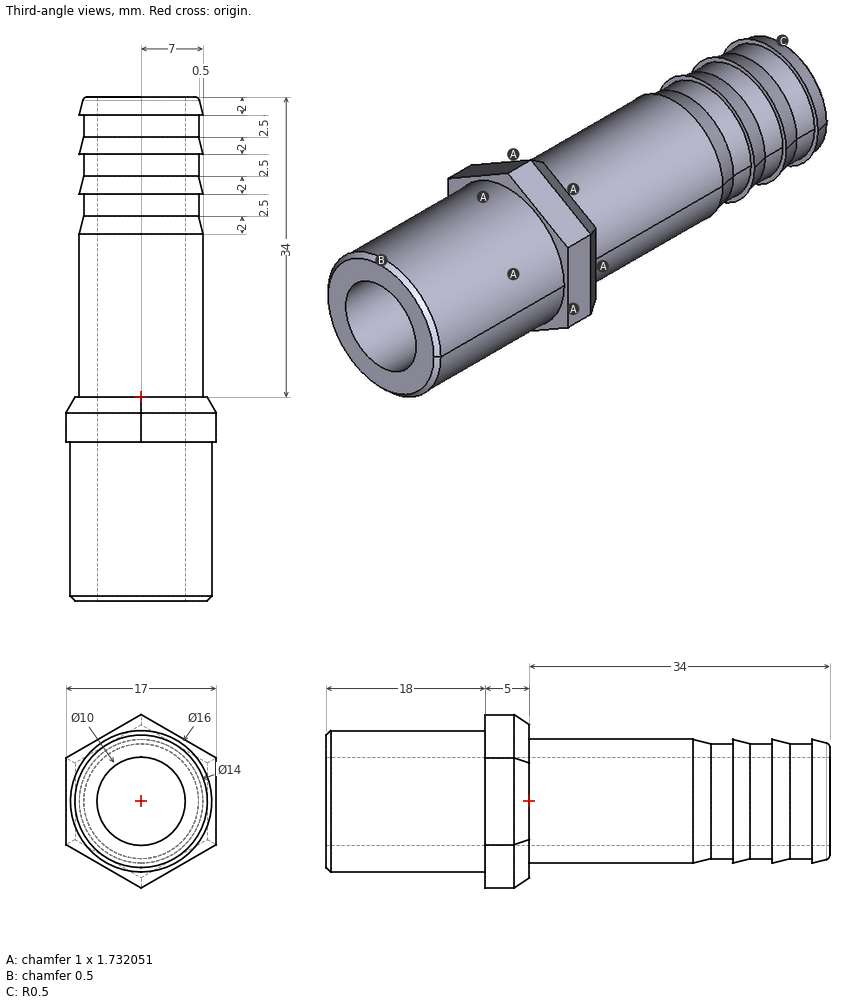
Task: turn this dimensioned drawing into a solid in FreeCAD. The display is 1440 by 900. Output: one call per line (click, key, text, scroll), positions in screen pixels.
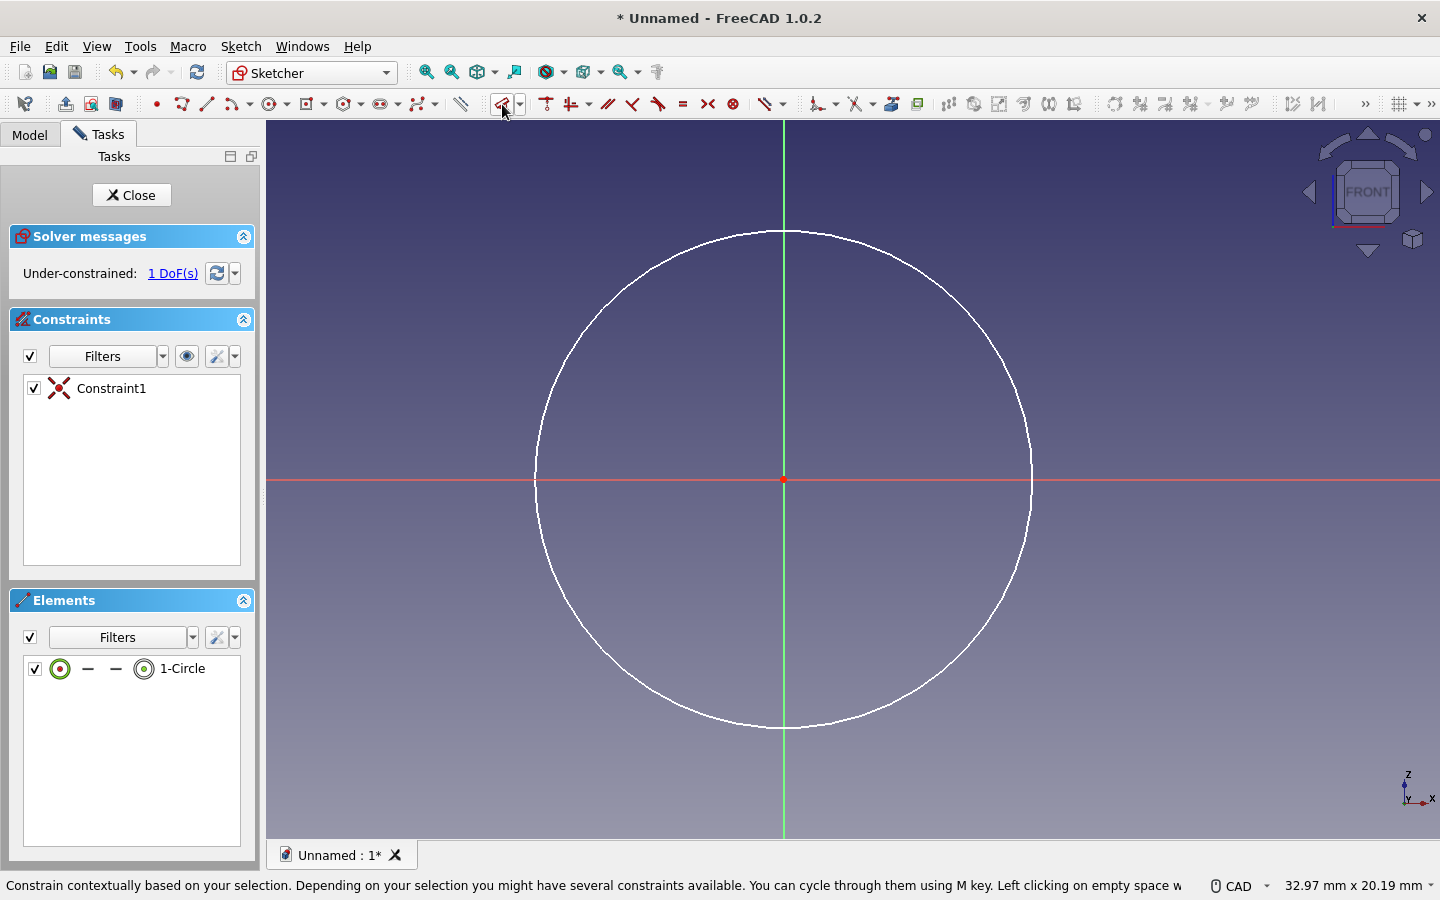
click(959, 303)
click(982, 280)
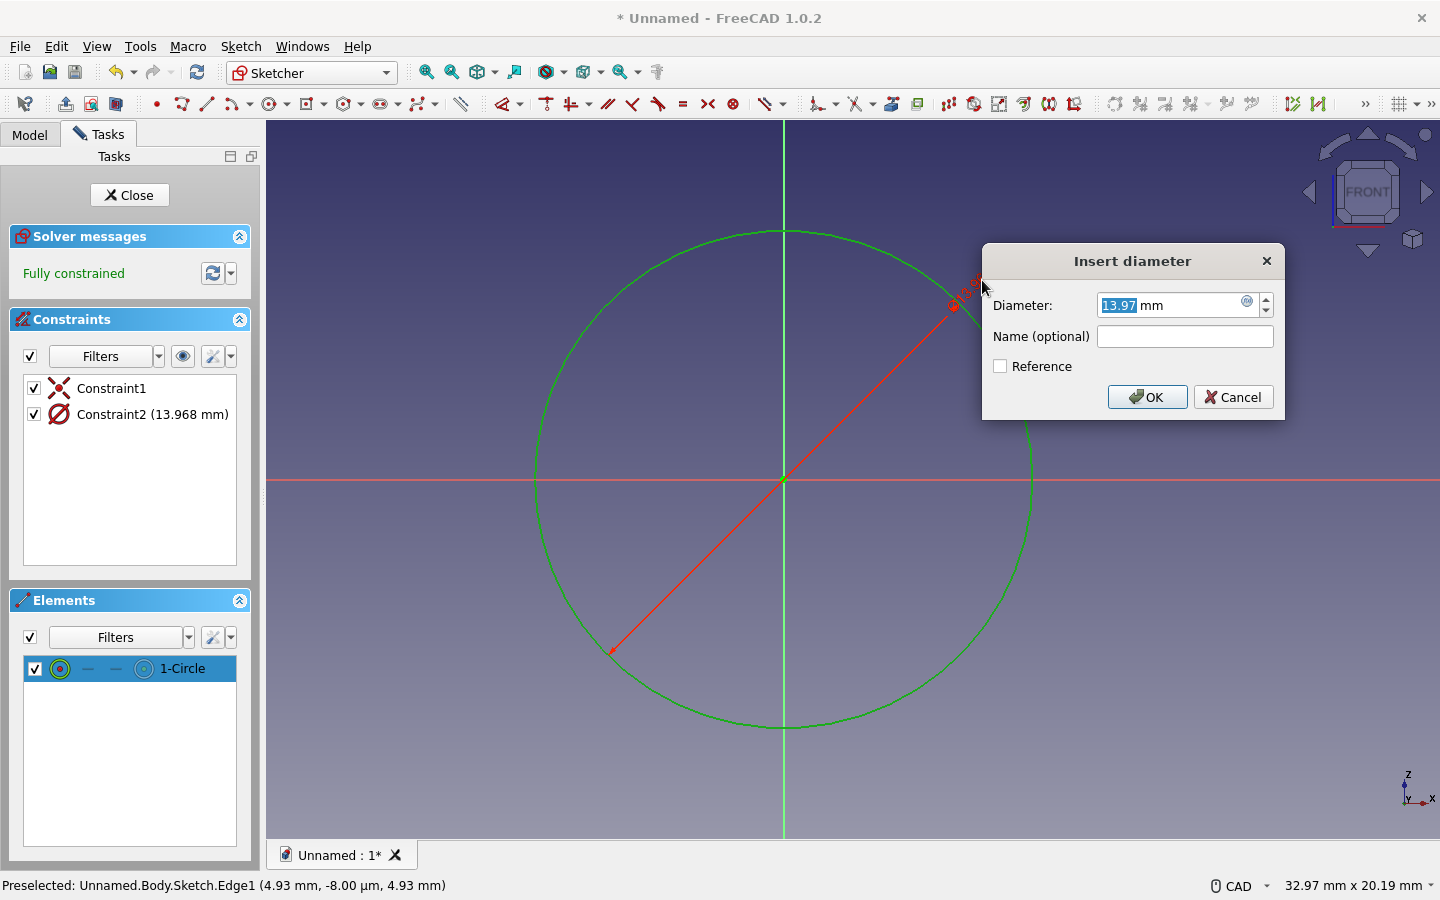
text(14)
key(Return)
key(Escape)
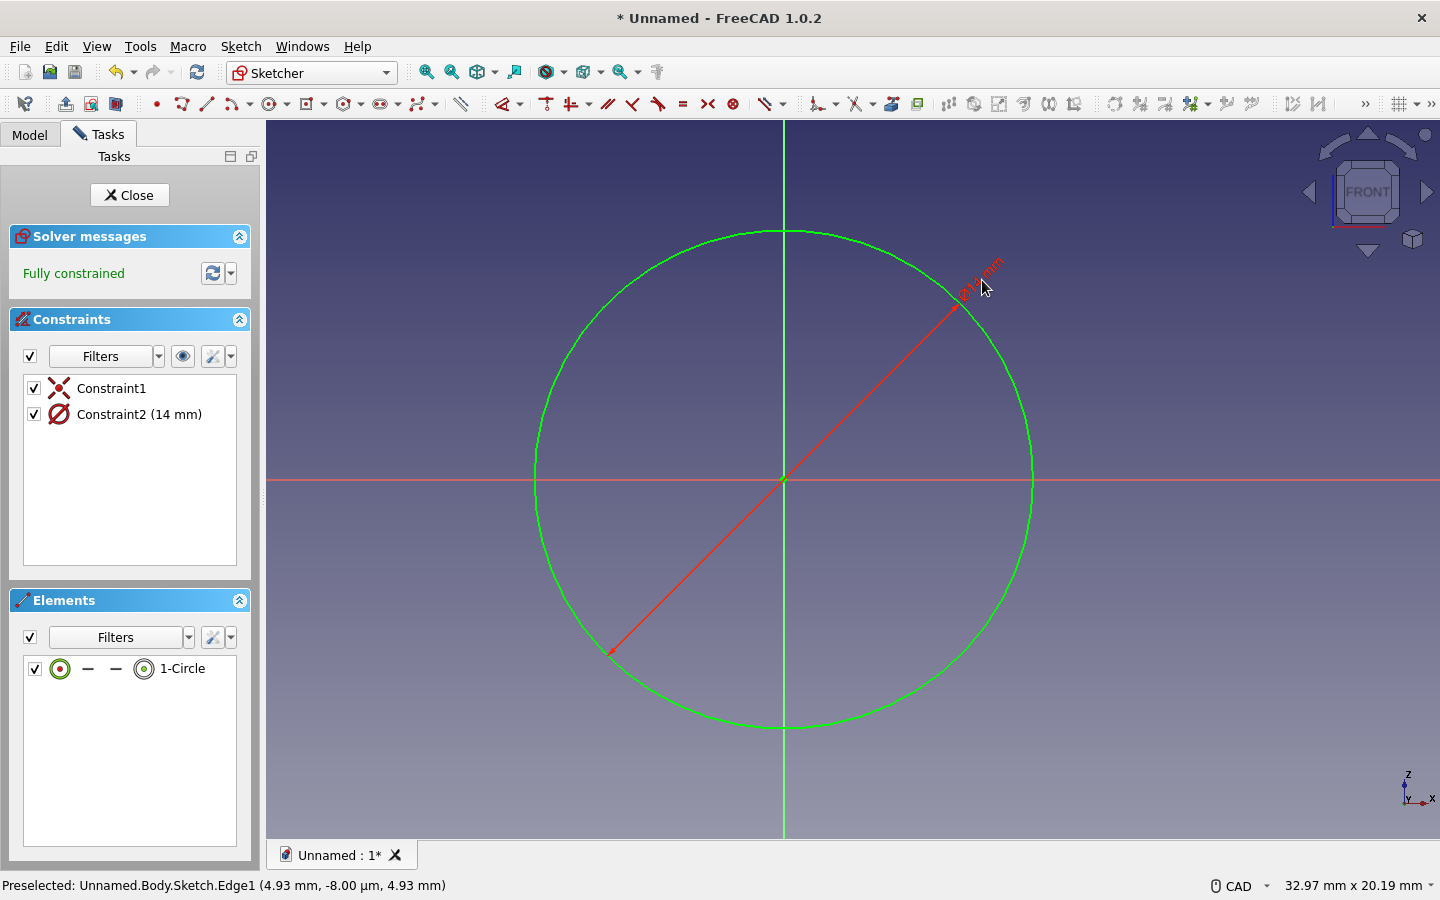
click(130, 195)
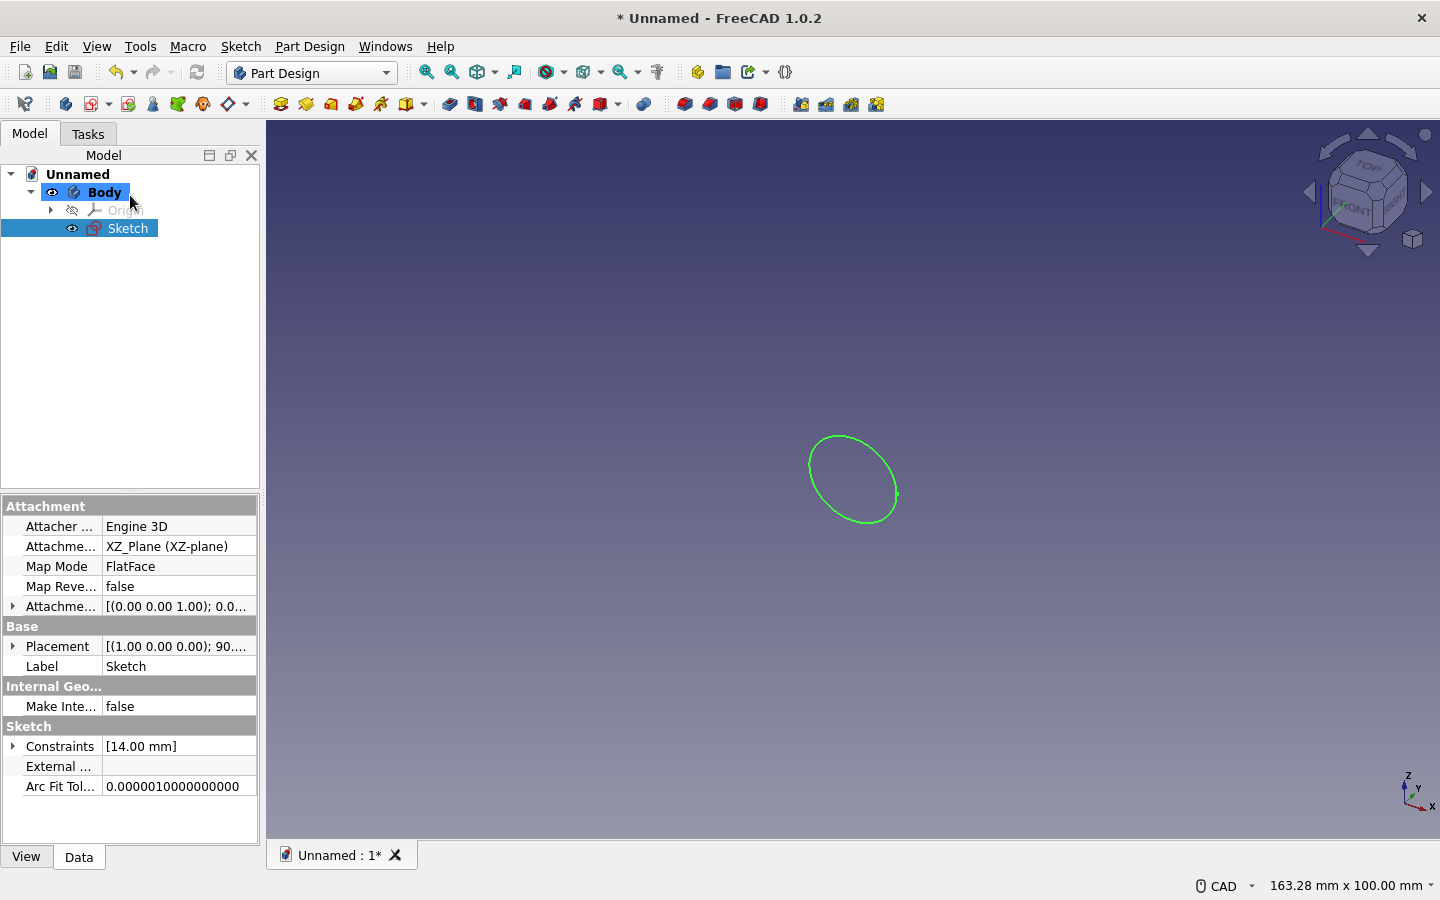
click(281, 104)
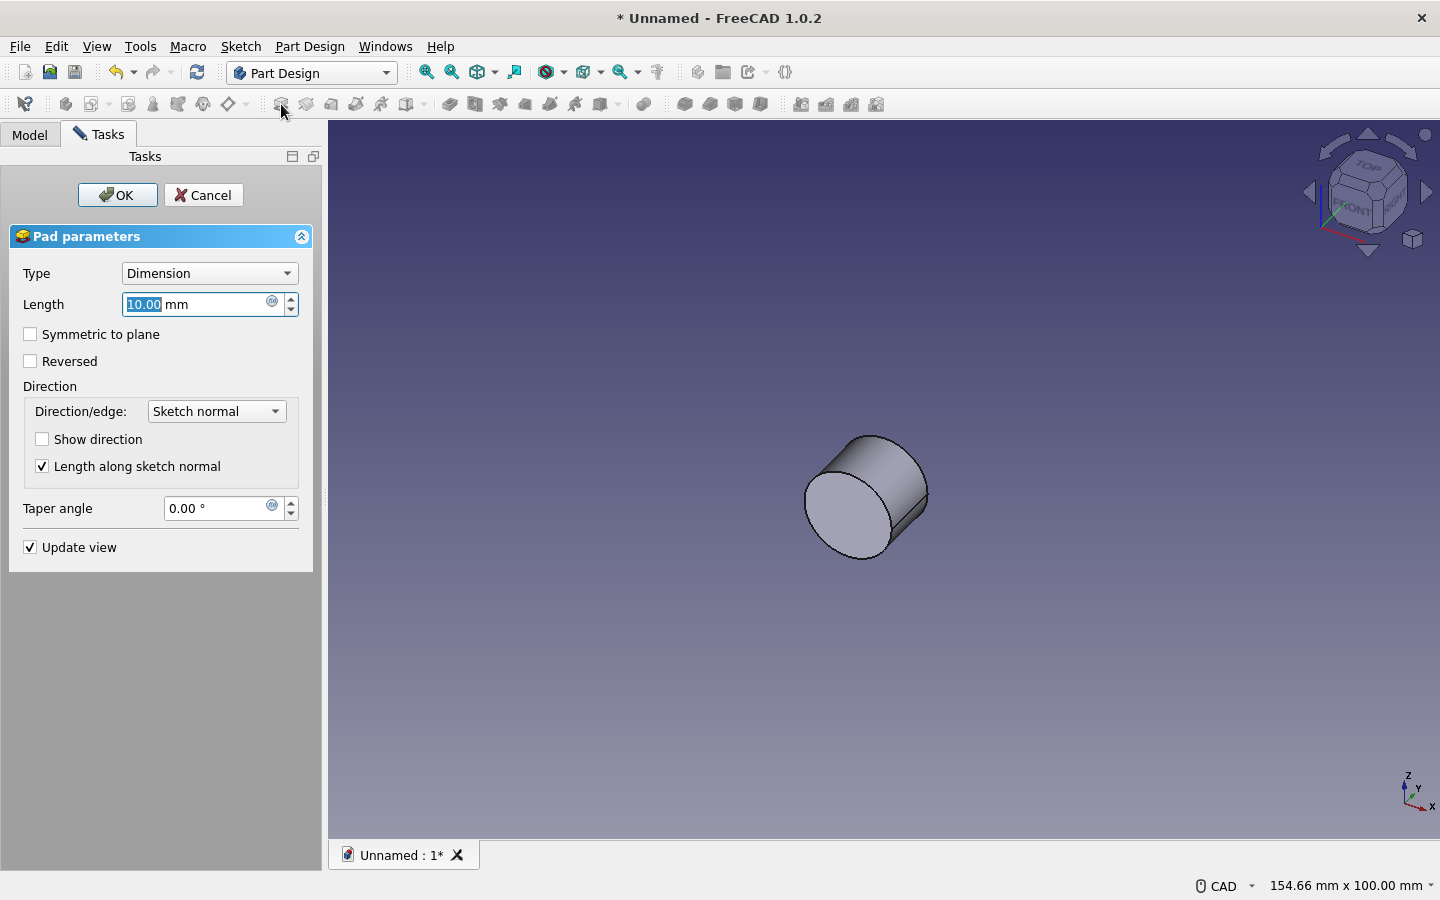
text(34)
key(Tab)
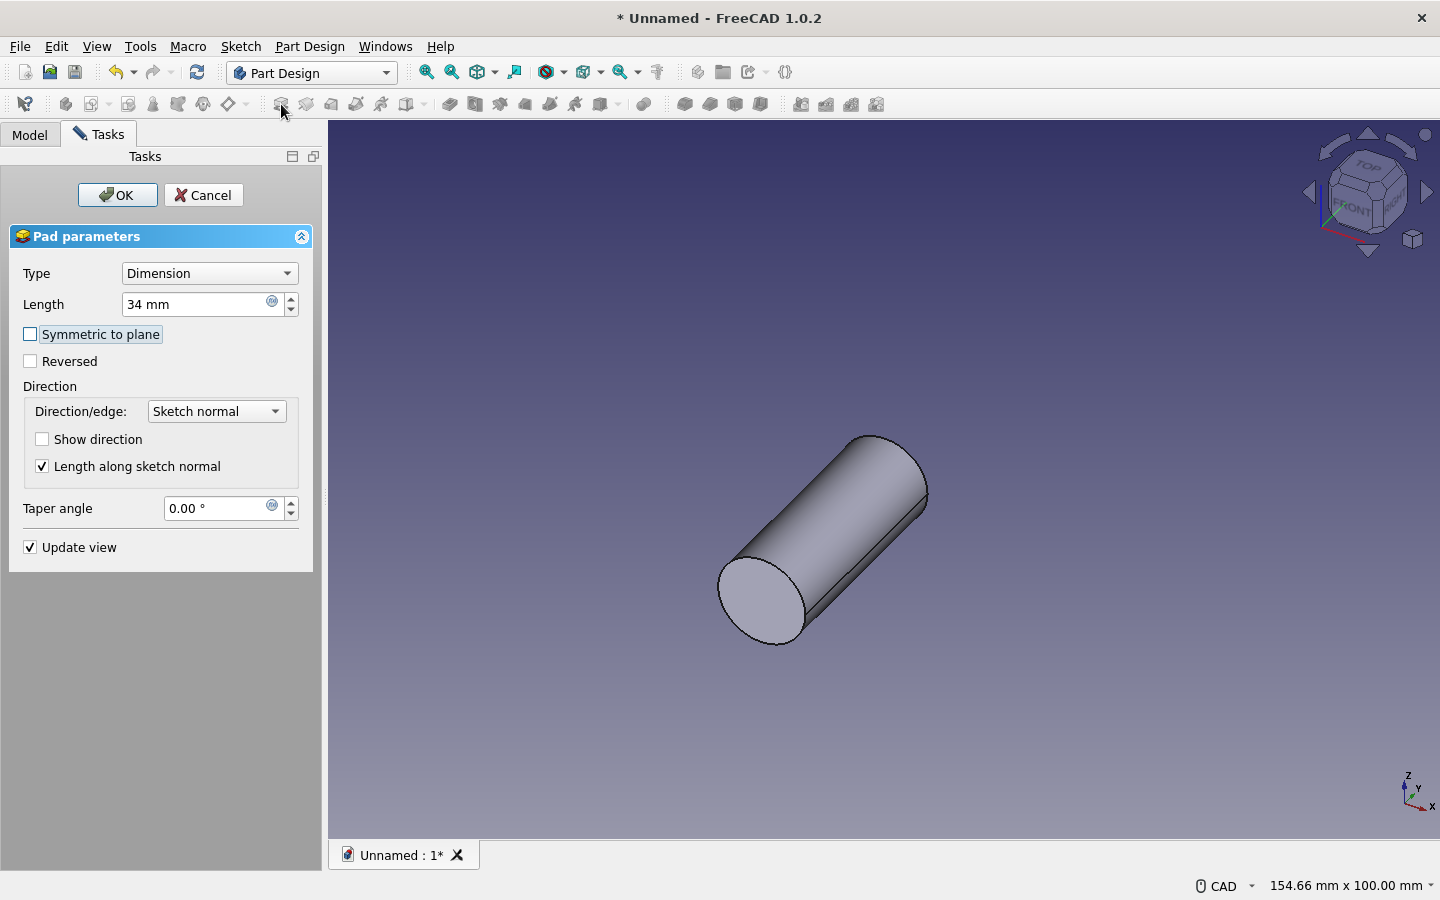
click(31, 361)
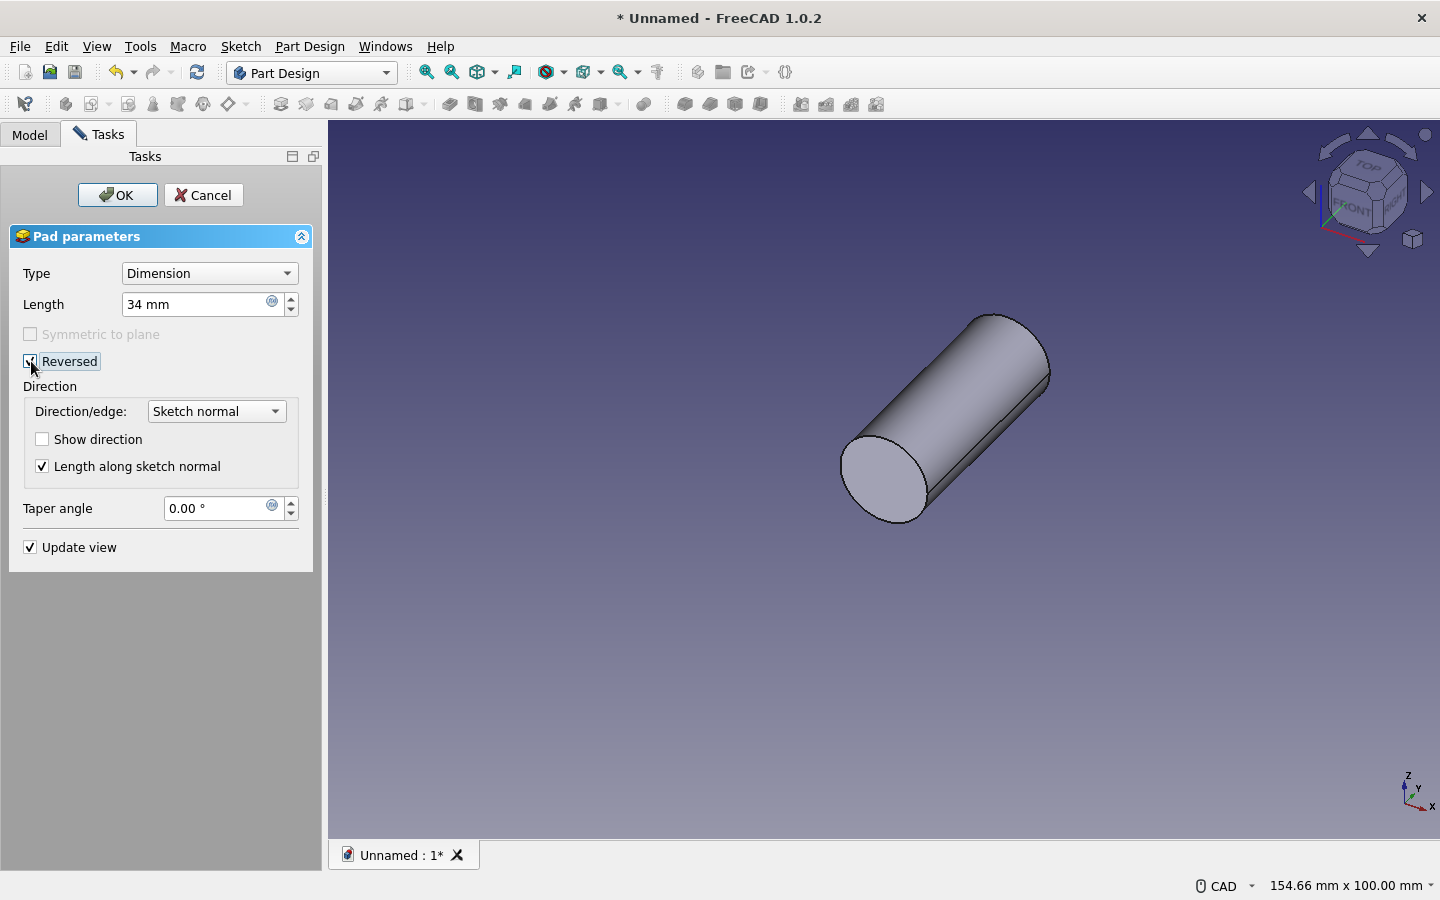
click(118, 195)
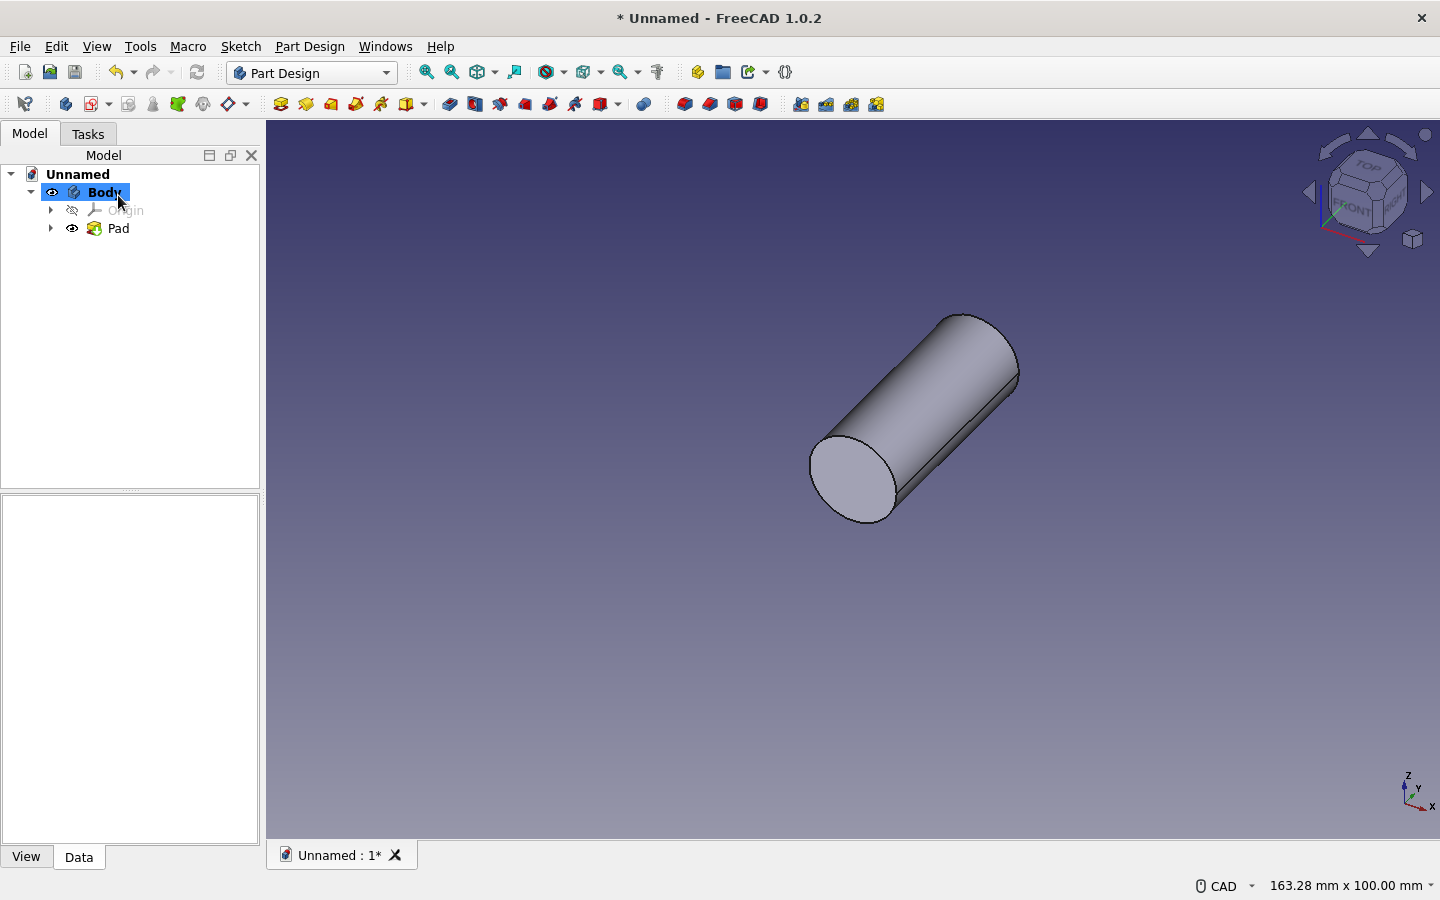
click(427, 72)